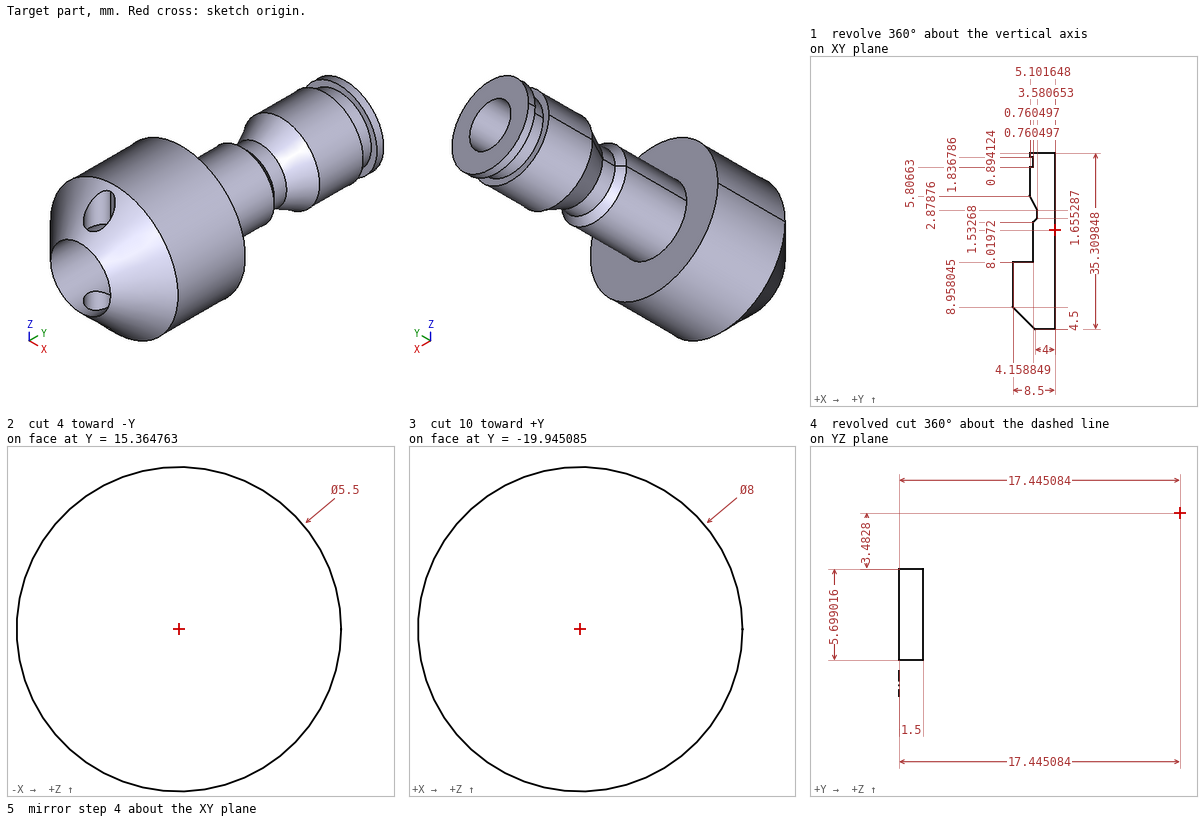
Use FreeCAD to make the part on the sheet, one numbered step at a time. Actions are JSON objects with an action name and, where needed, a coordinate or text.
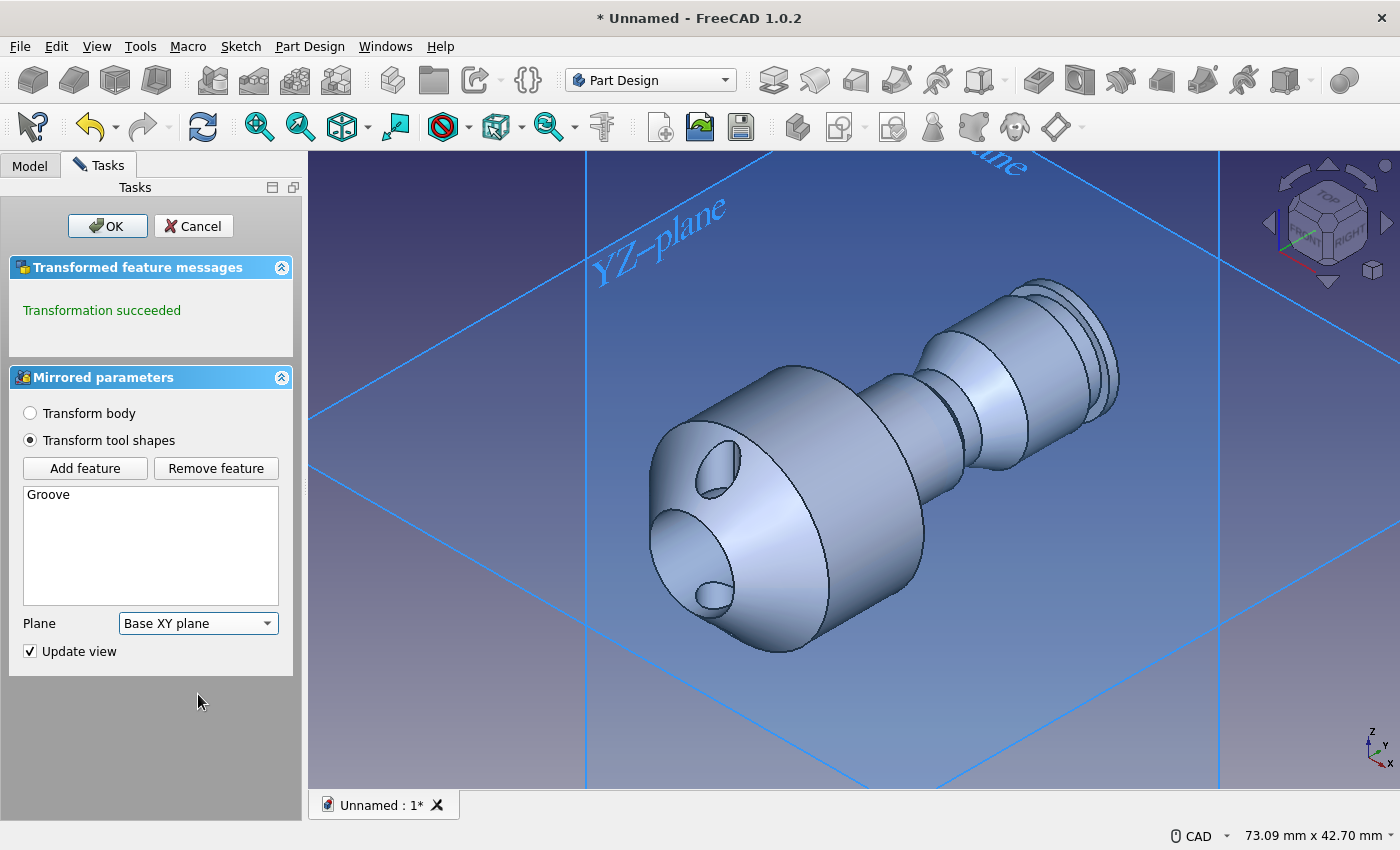
{"action": "left_click", "coordinate": [108, 226]}